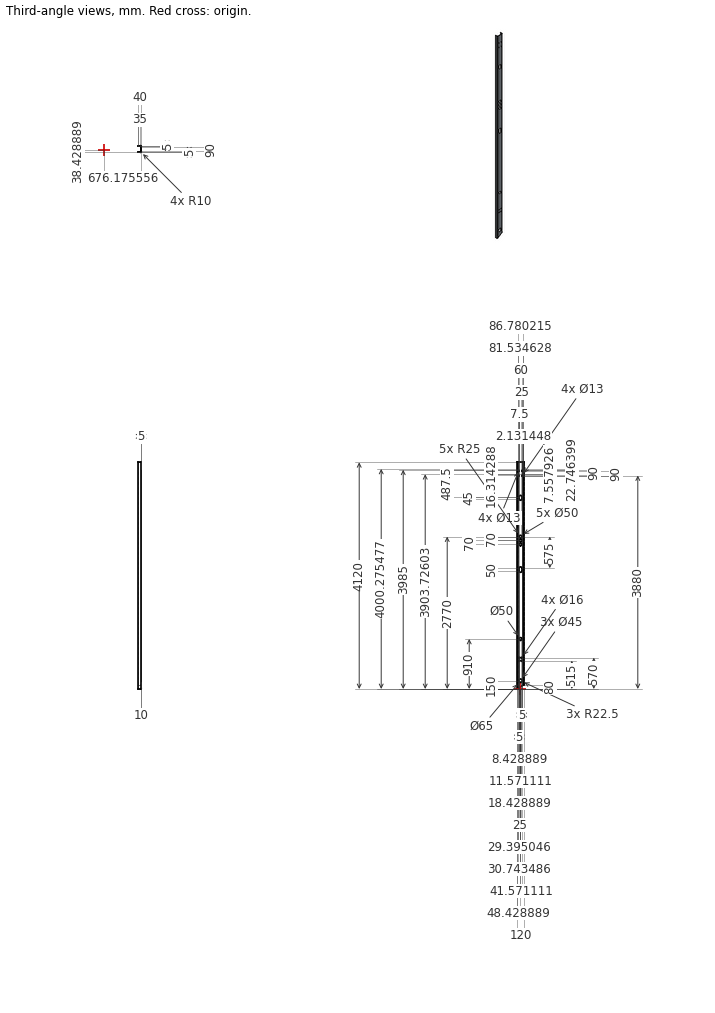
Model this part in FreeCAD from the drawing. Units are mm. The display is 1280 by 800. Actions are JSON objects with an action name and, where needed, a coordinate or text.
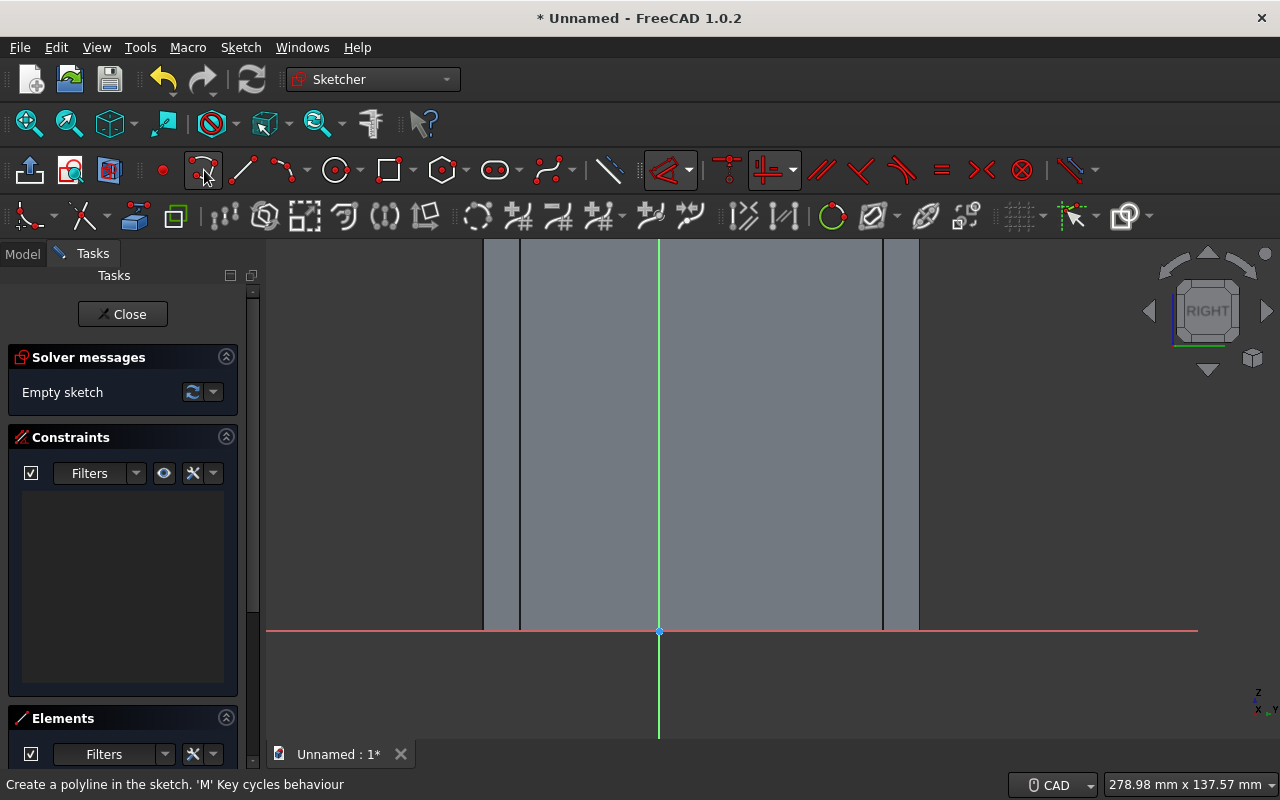
{"action": "left_click", "coordinate": [483, 631]}
{"action": "left_click", "coordinate": [919, 622]}
{"action": "left_click", "coordinate": [919, 341]}
{"action": "left_click", "coordinate": [483, 631]}
{"action": "key", "text": "Escape"}
{"action": "key", "text": "Escape"}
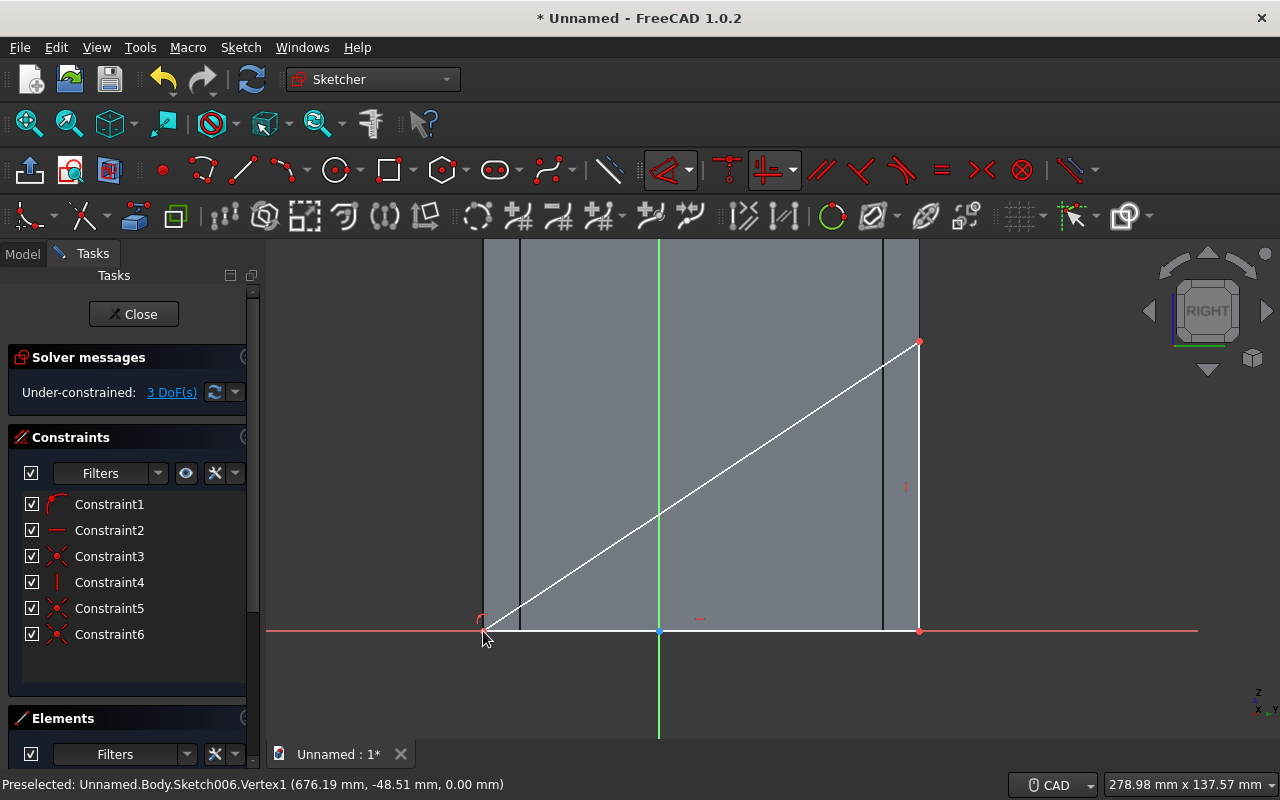
{"action": "left_click", "coordinate": [919, 545]}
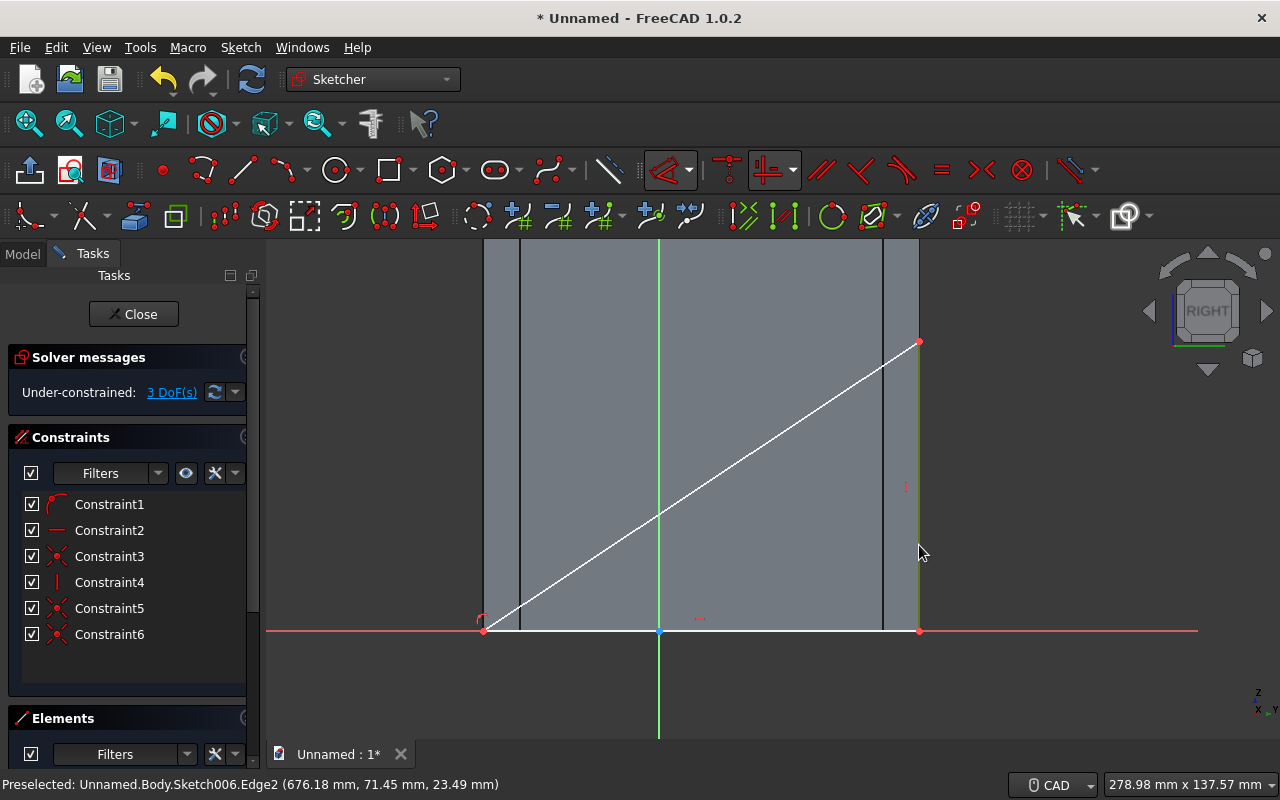
{"action": "key", "text": "i"}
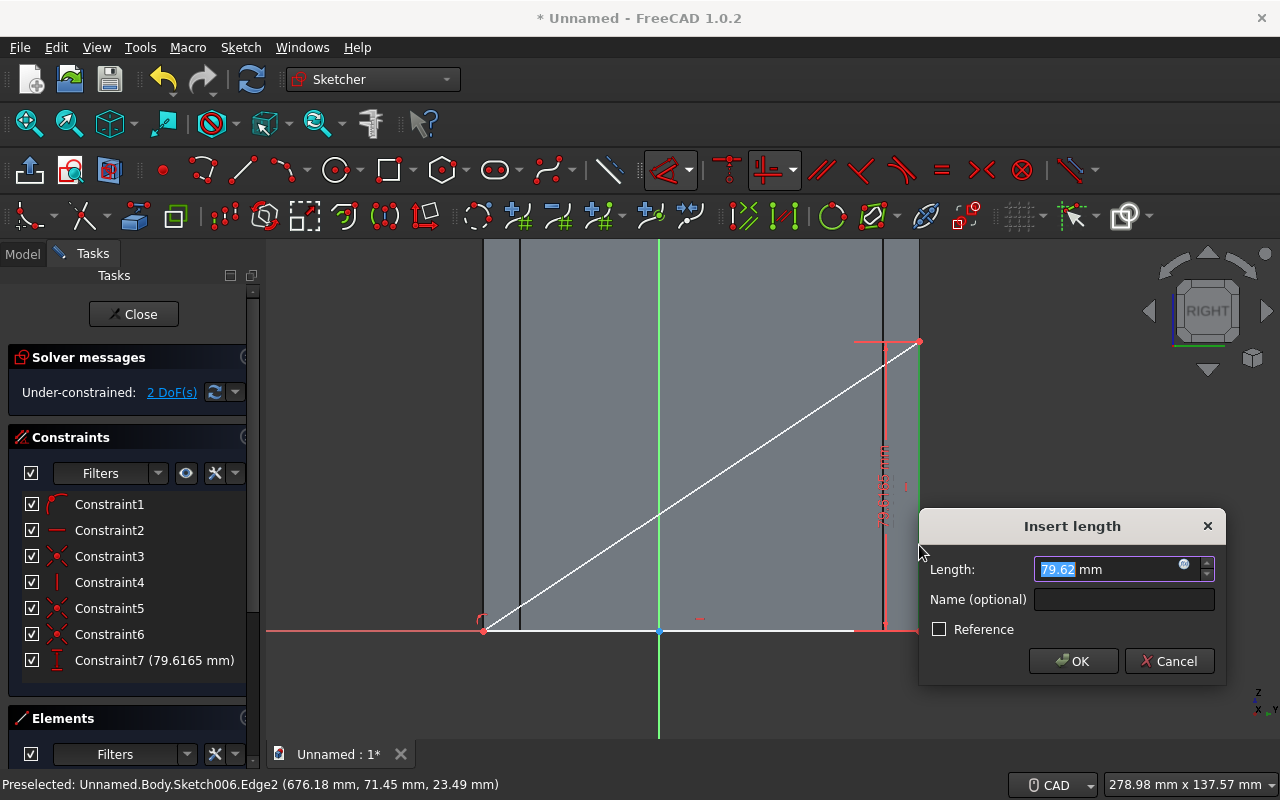
{"action": "type", "text": "80"}
{"action": "key", "text": "Return"}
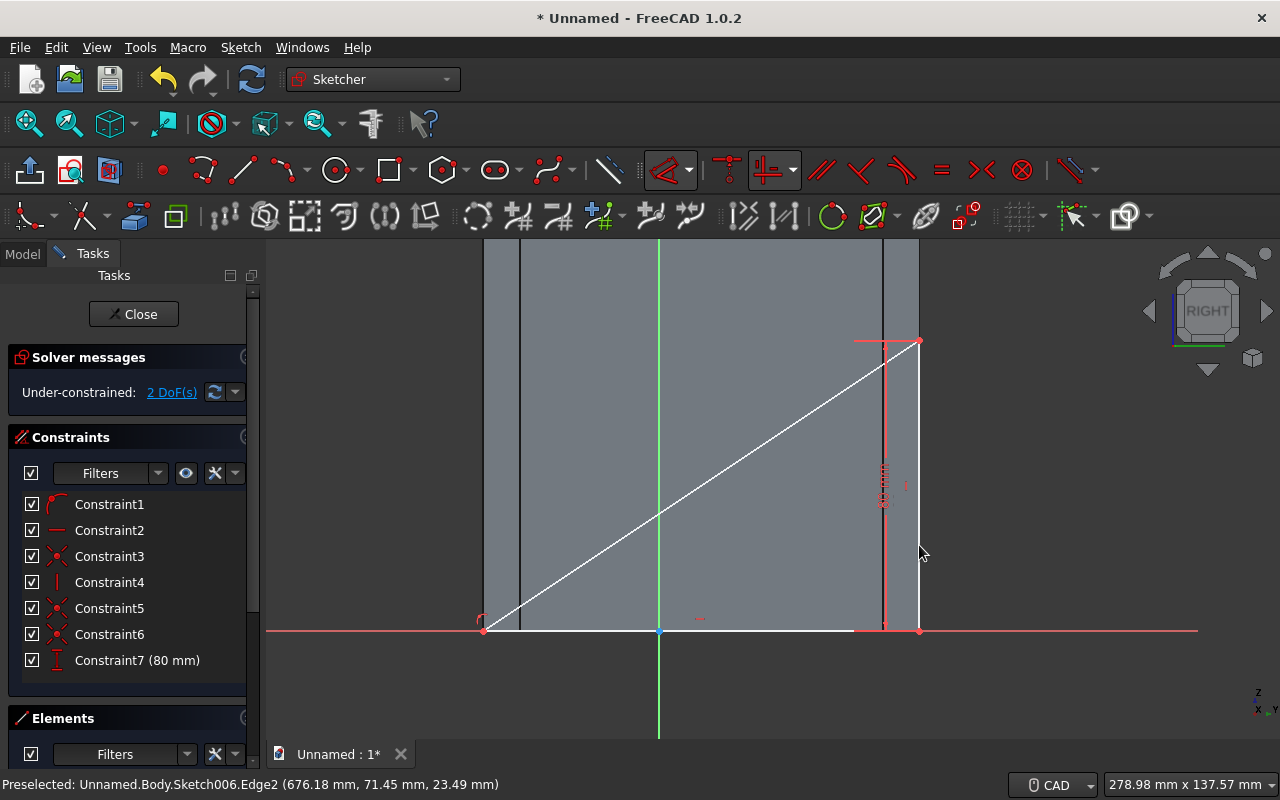
{"action": "left_click", "coordinate": [614, 631]}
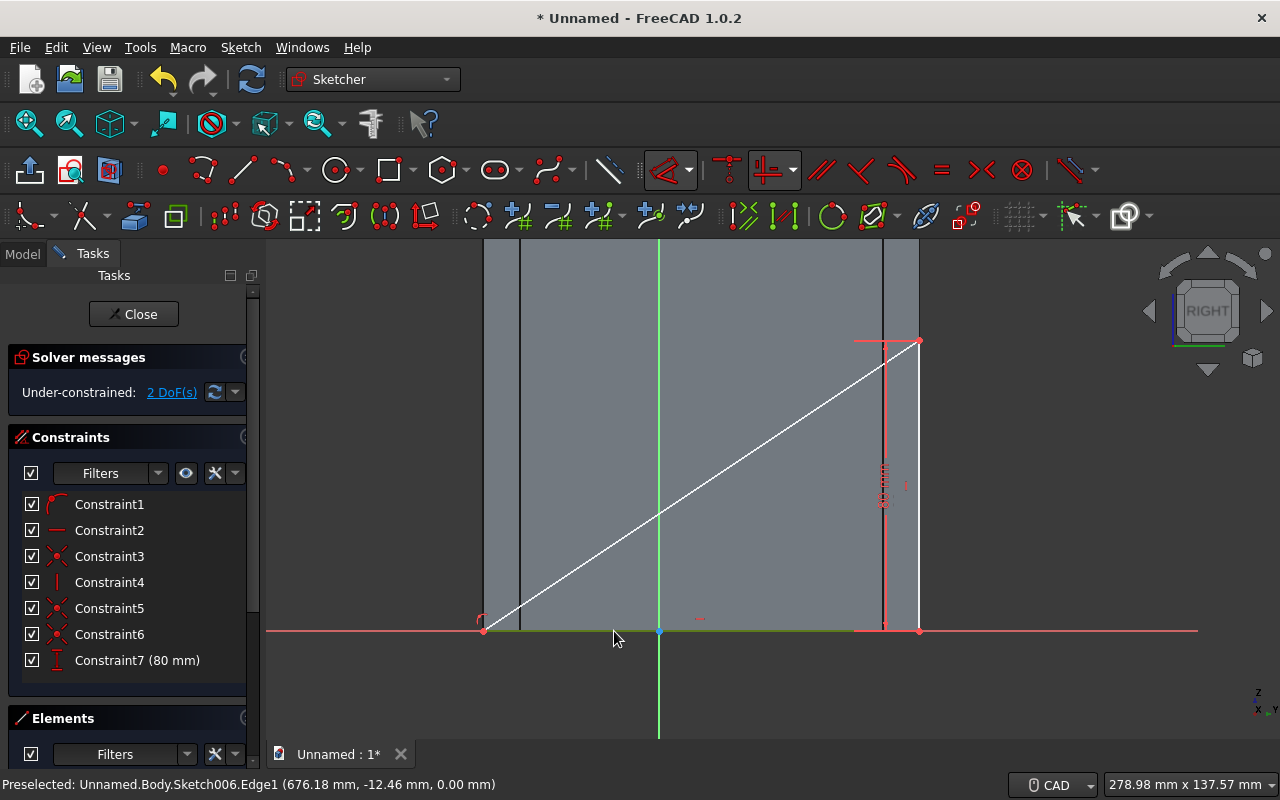
{"action": "key", "text": "l"}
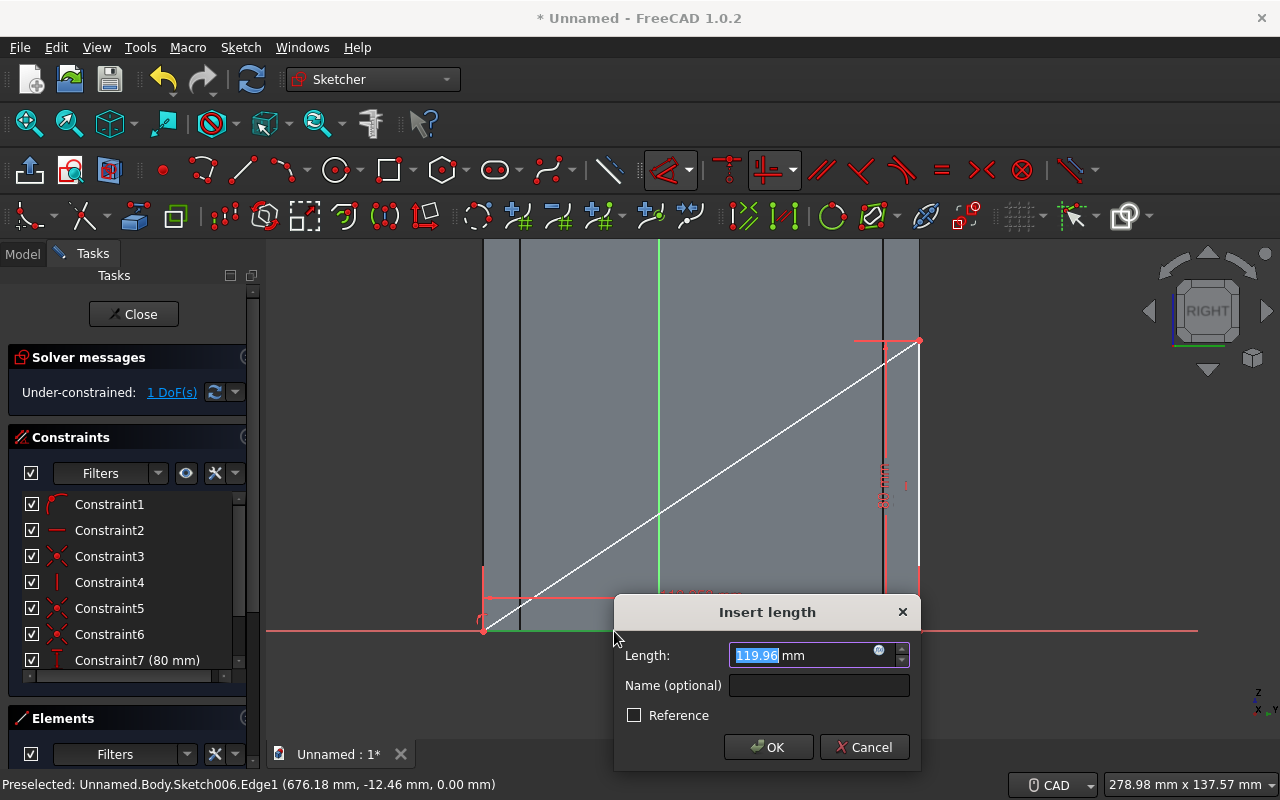
{"action": "type", "text": "120"}
{"action": "key", "text": "Return"}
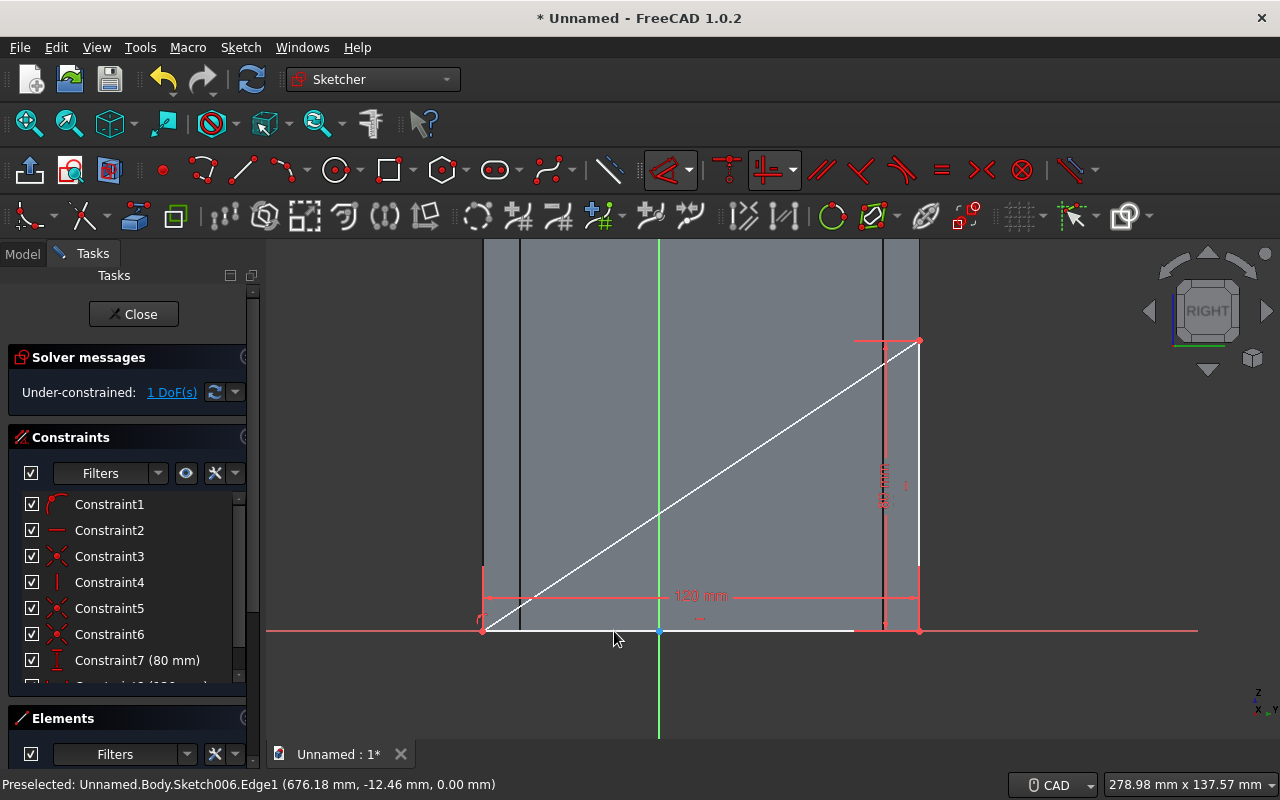
{"action": "left_click", "coordinate": [483, 631]}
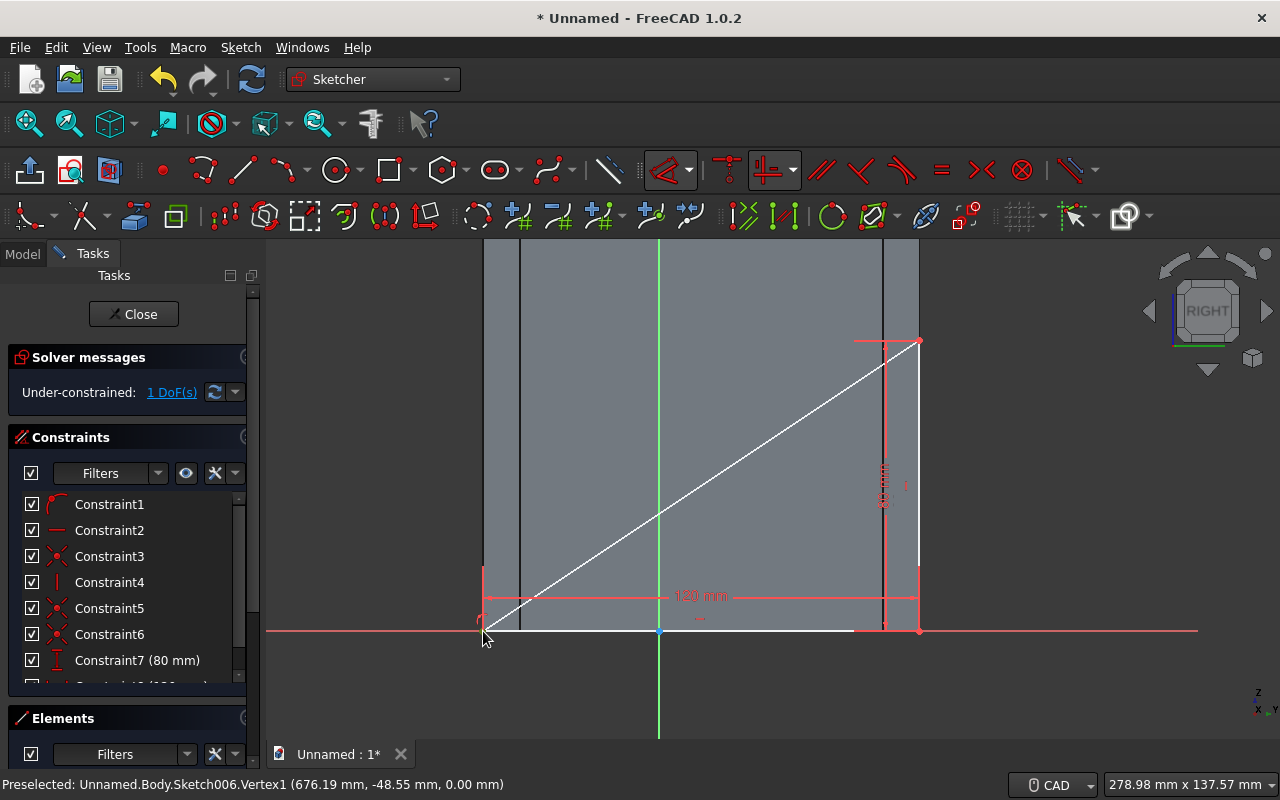
{"action": "key", "text": "l"}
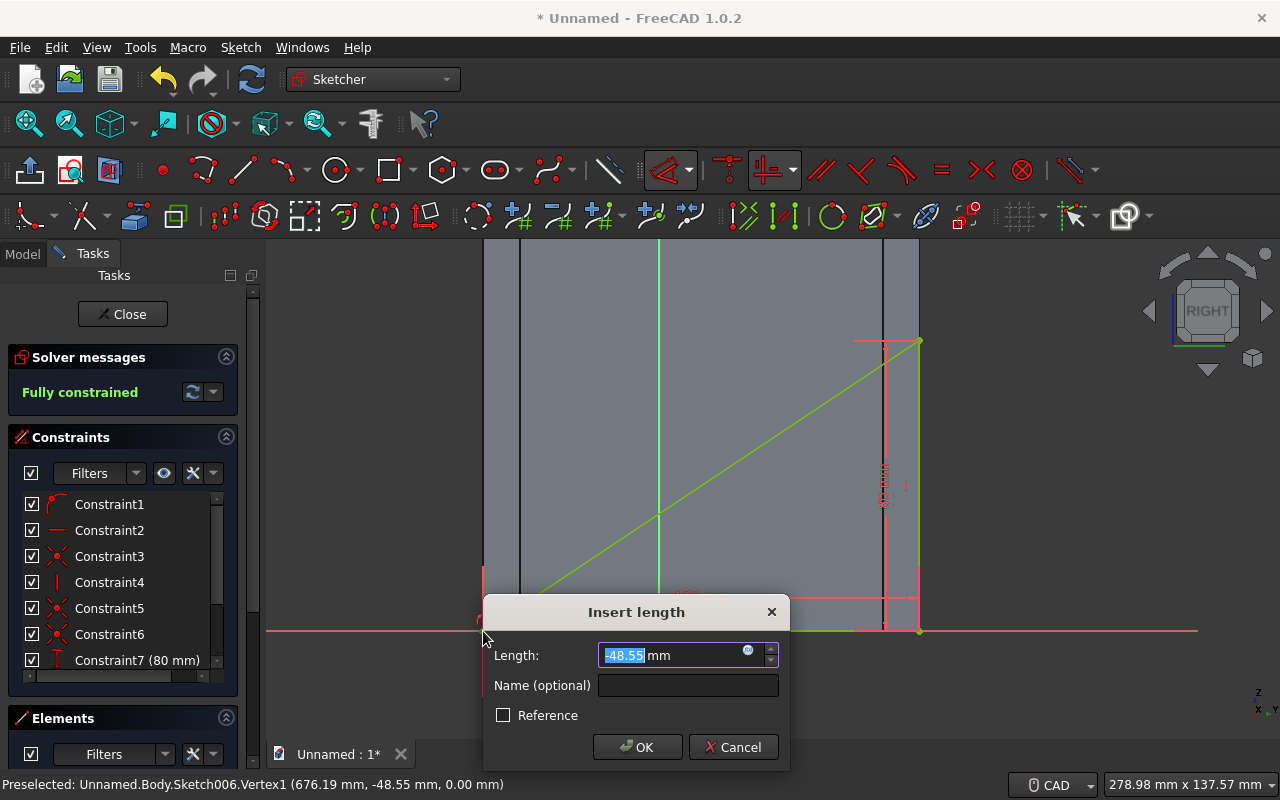
{"action": "type", "text": "-48.428889"}
{"action": "key", "text": "Return"}